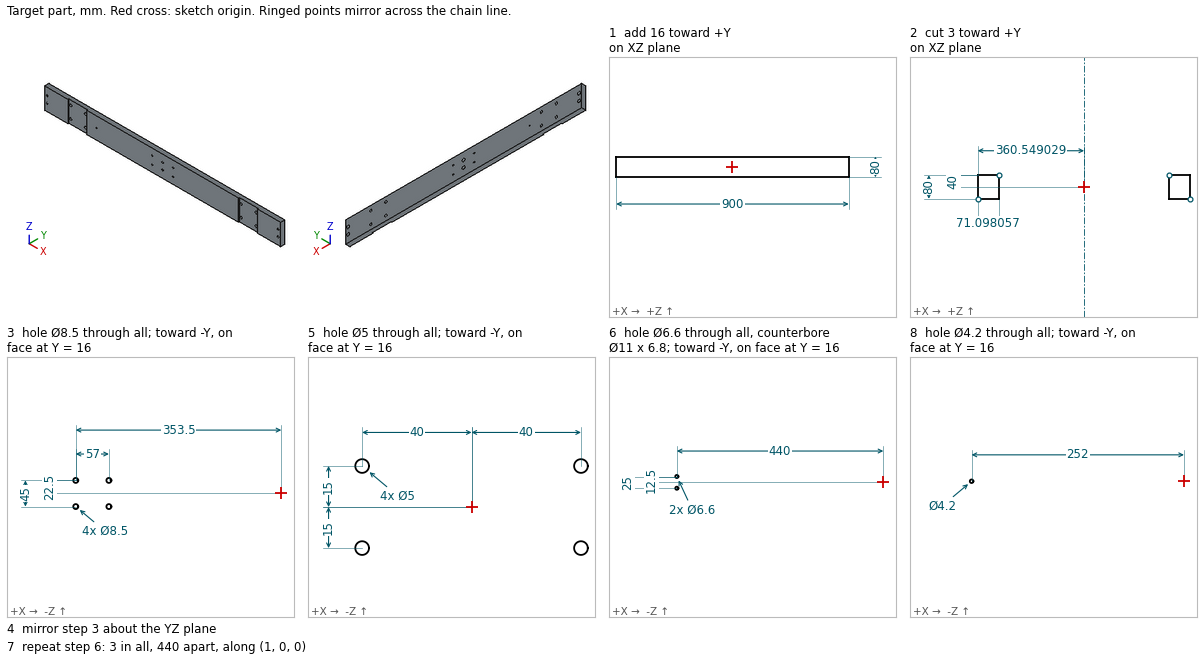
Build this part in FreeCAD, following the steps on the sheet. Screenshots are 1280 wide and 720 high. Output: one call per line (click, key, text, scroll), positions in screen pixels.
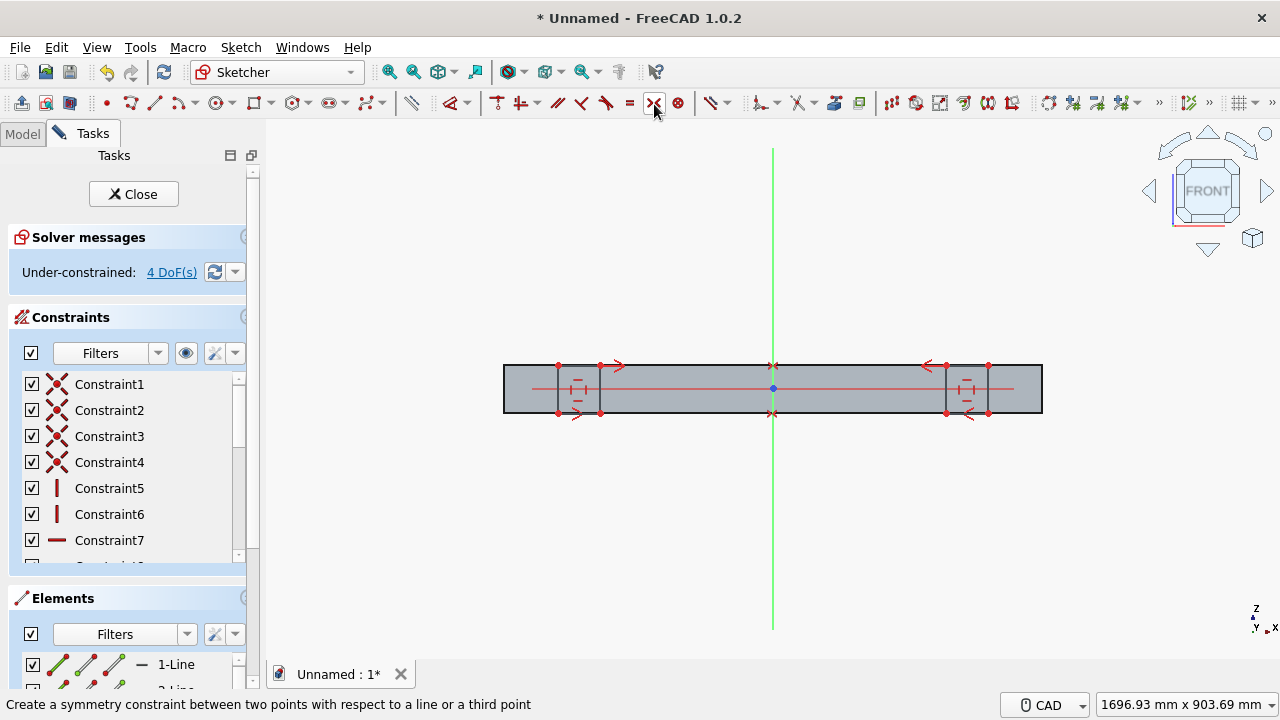
click(450, 104)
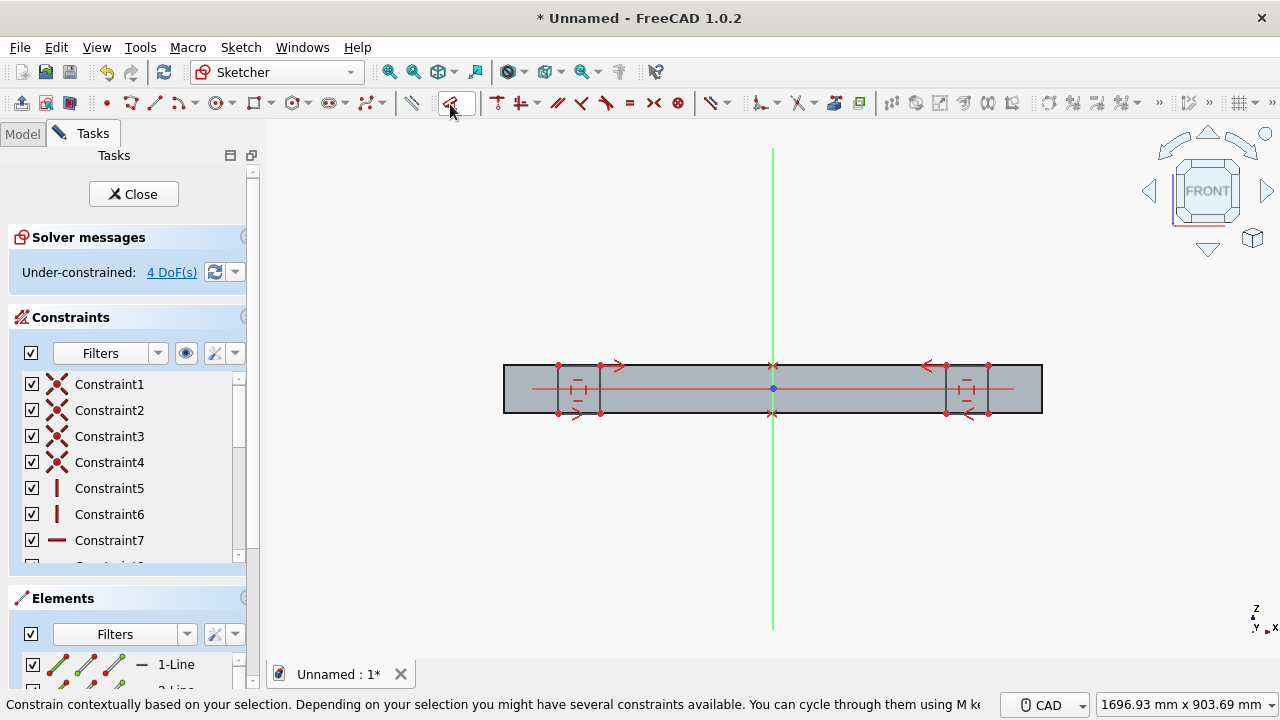
scroll(558, 400, up, 2)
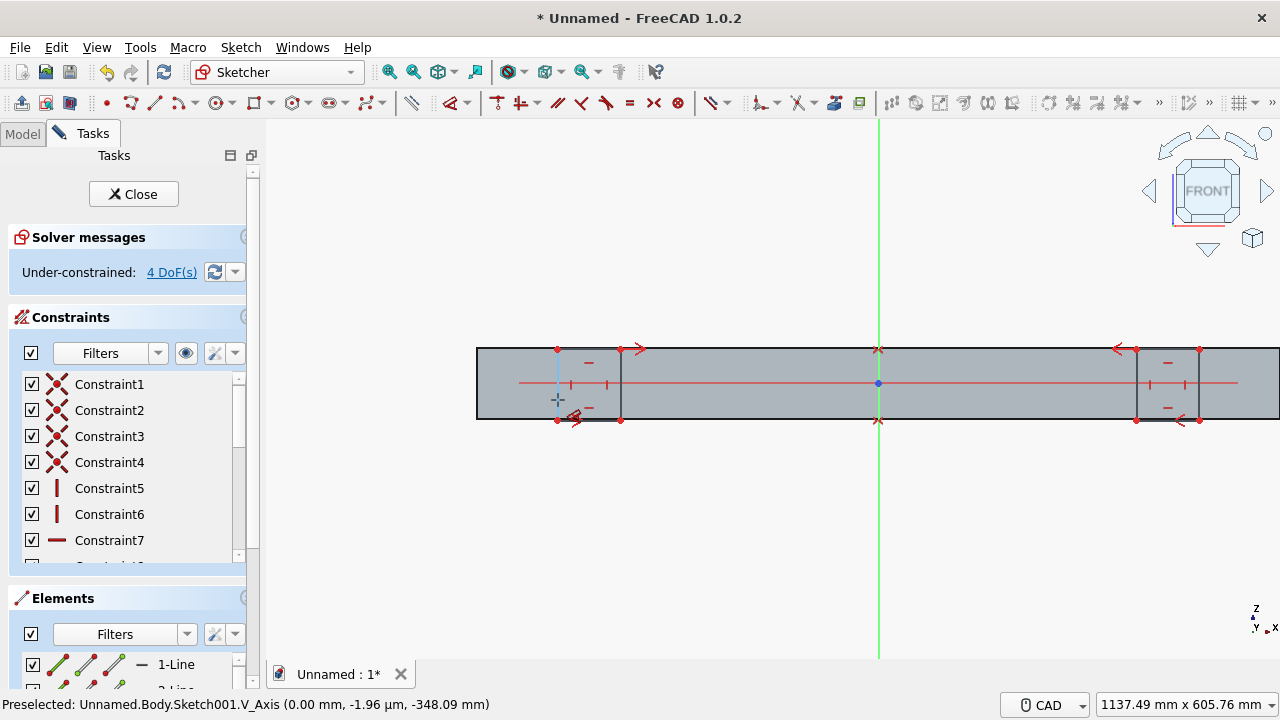
click(558, 399)
click(524, 368)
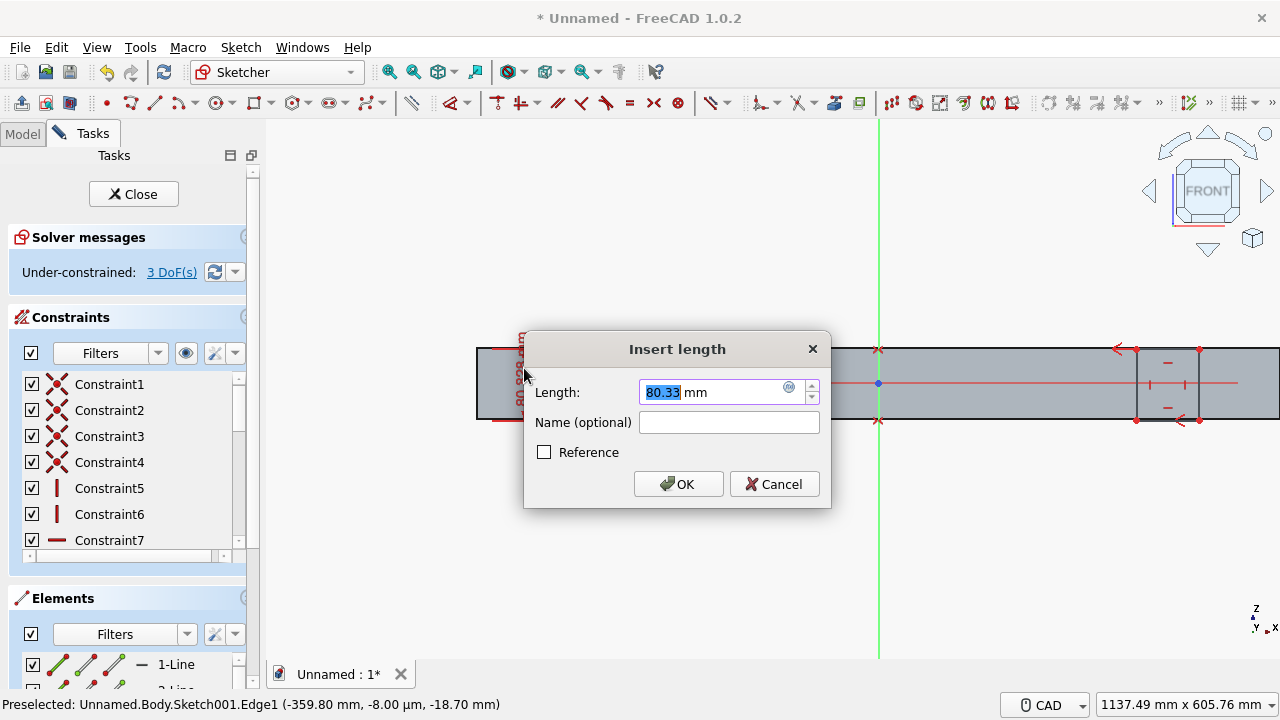
text(80)
key(Return)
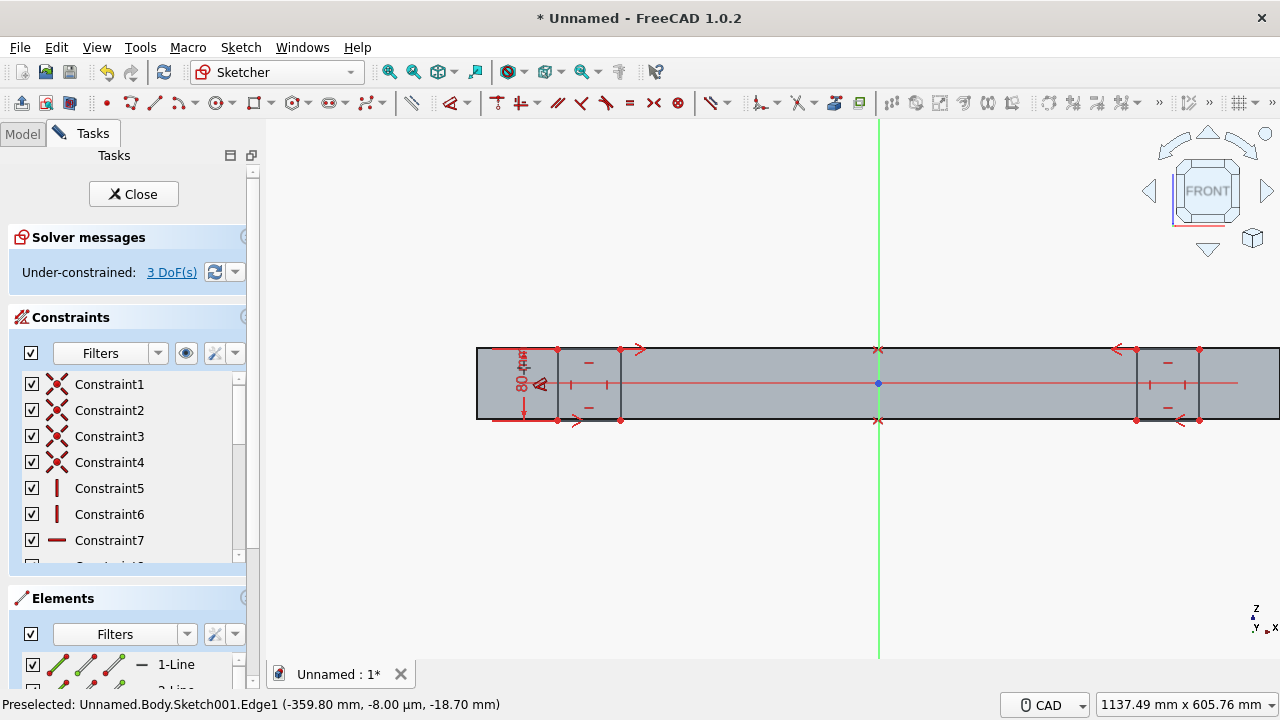
click(558, 349)
click(913, 366)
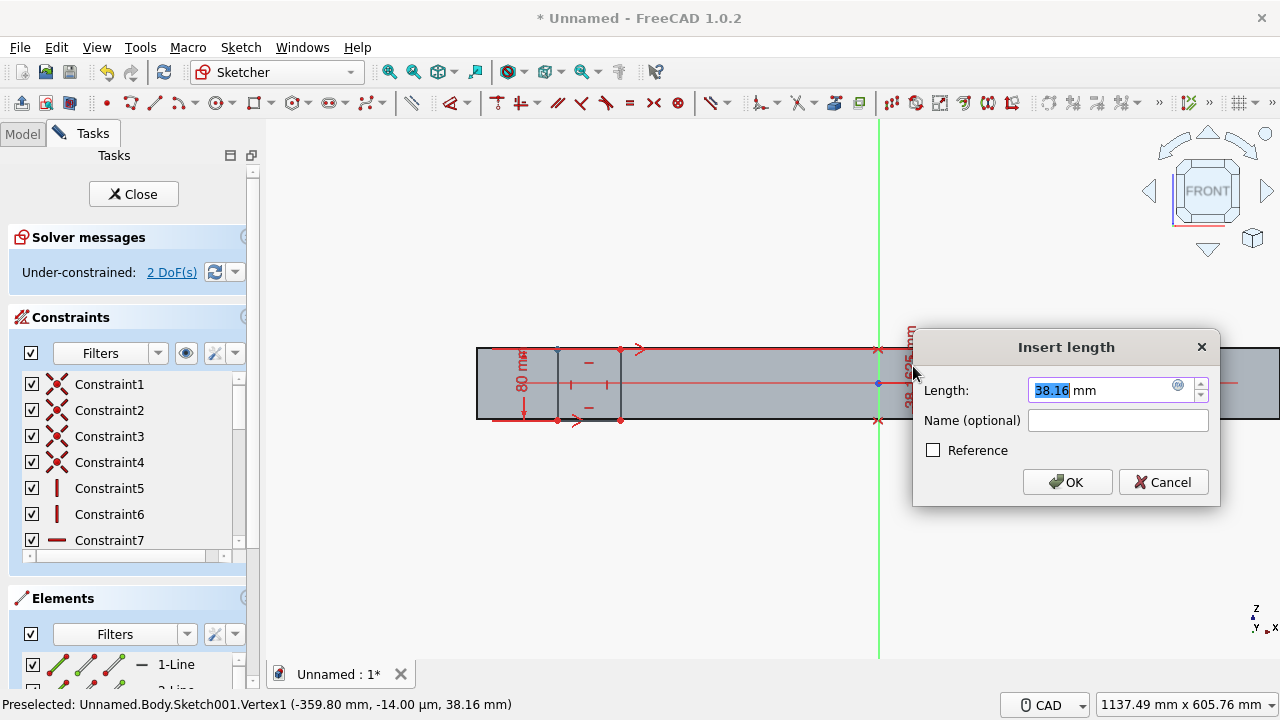
text(40)
key(Return)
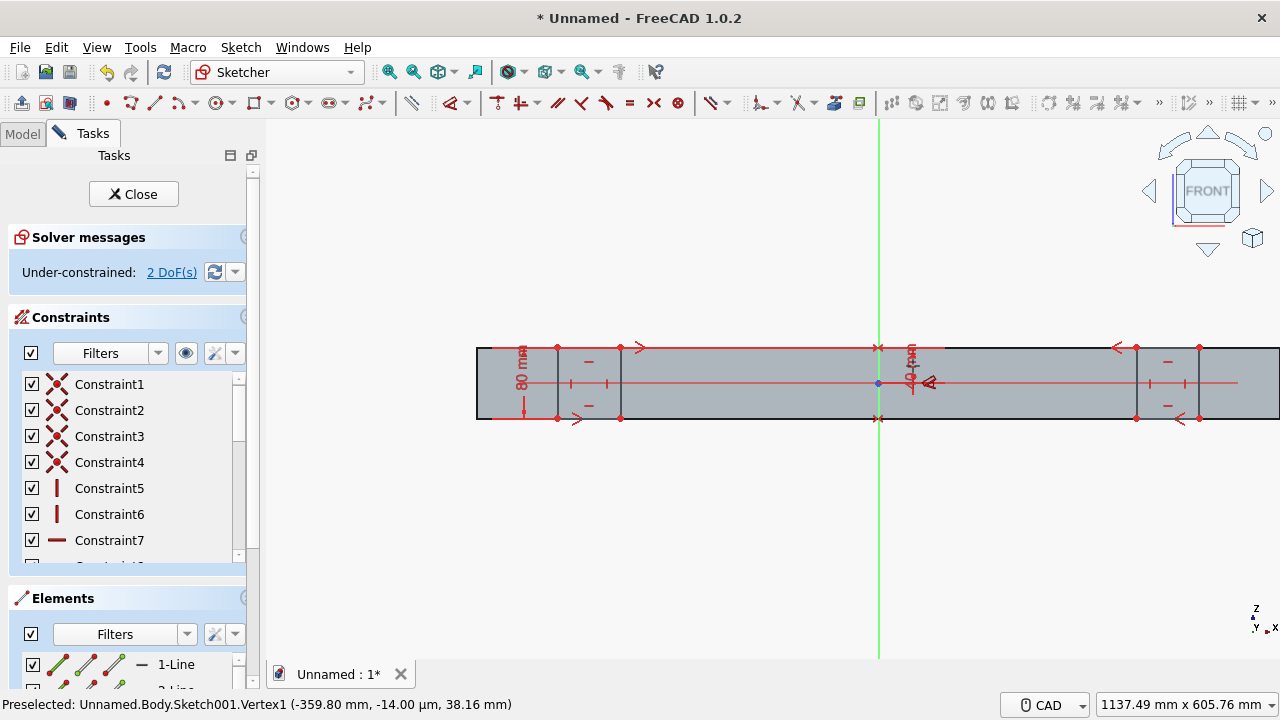
click(577, 419)
click(589, 453)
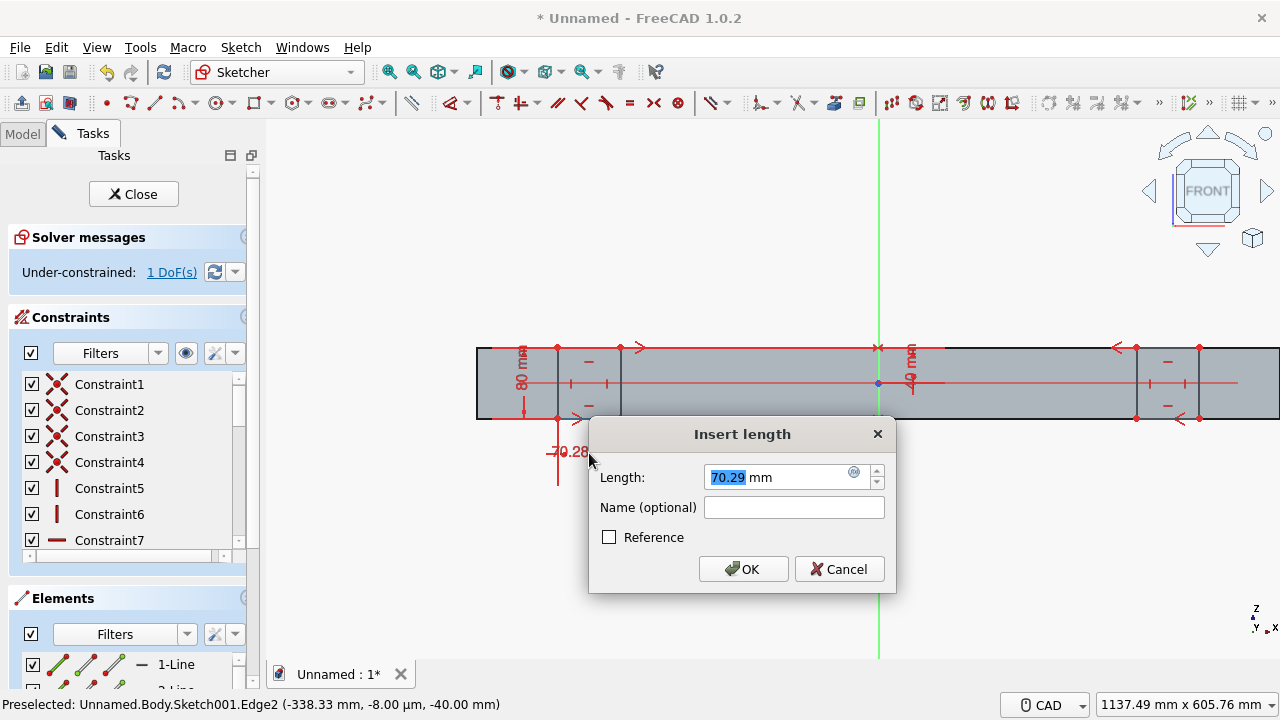
text(71.098057)
key(Return)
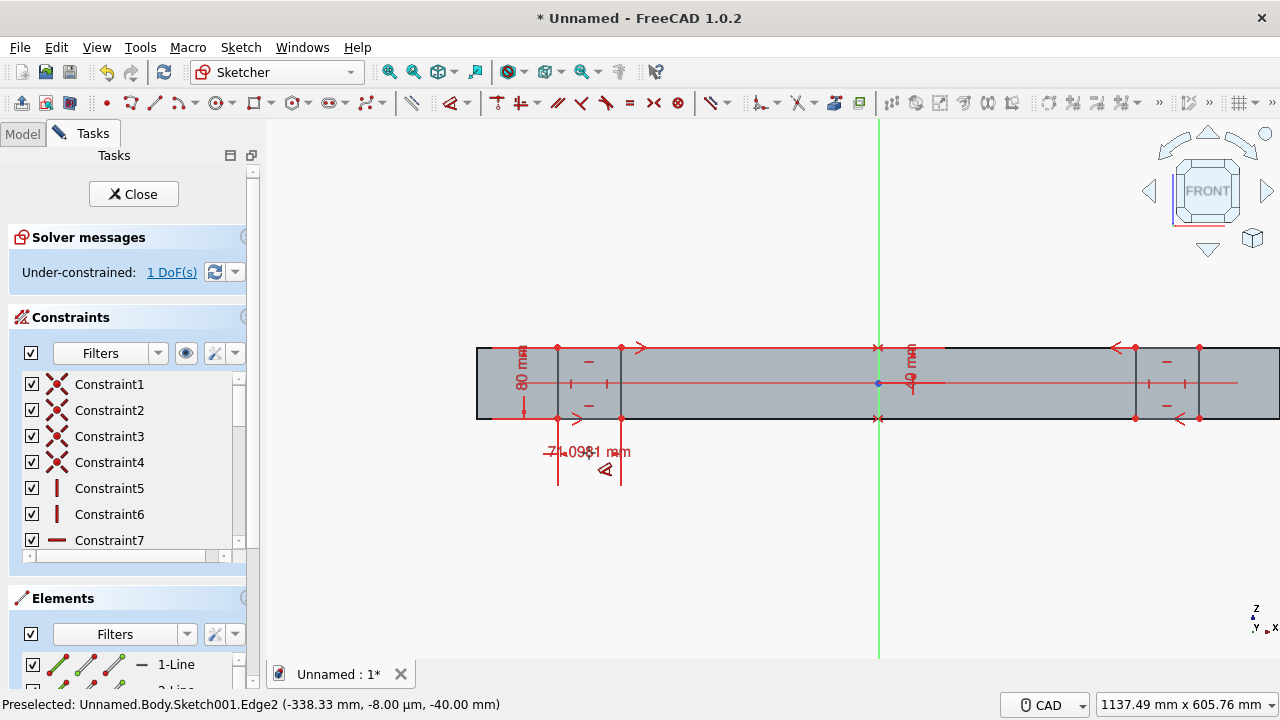
click(558, 348)
click(718, 314)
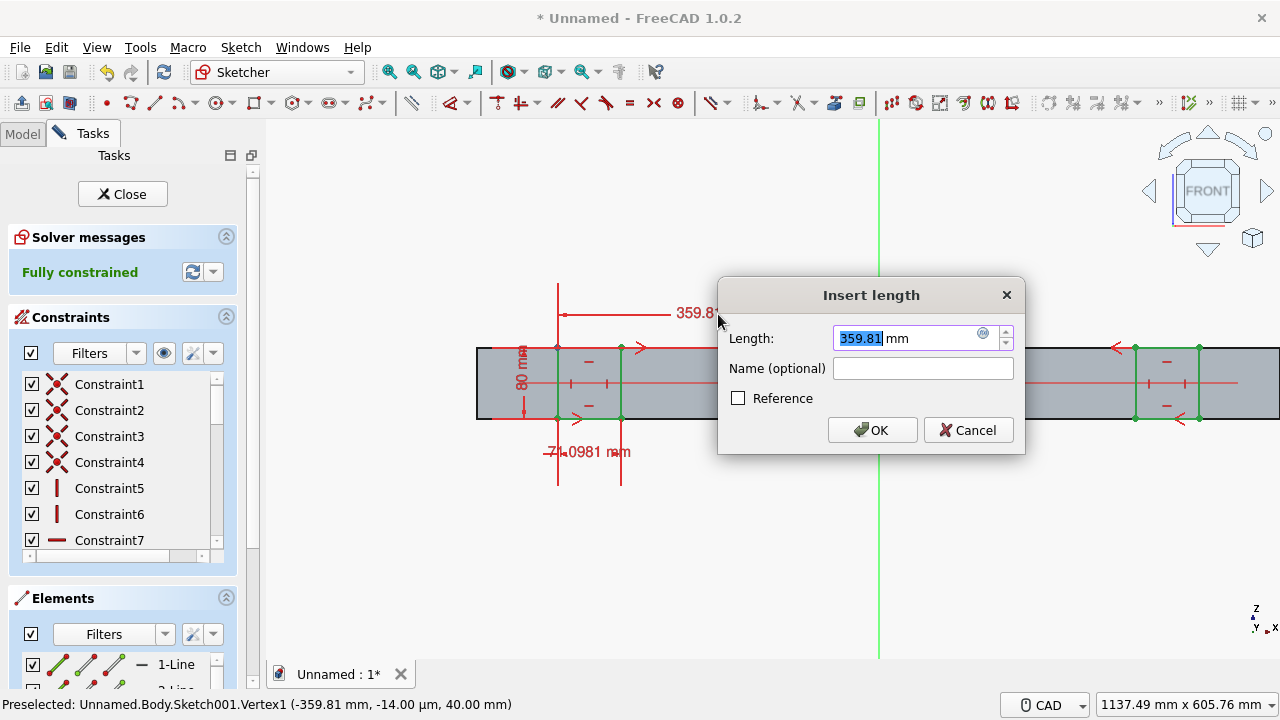
text(360.549029)
key(Return)
key(Escape)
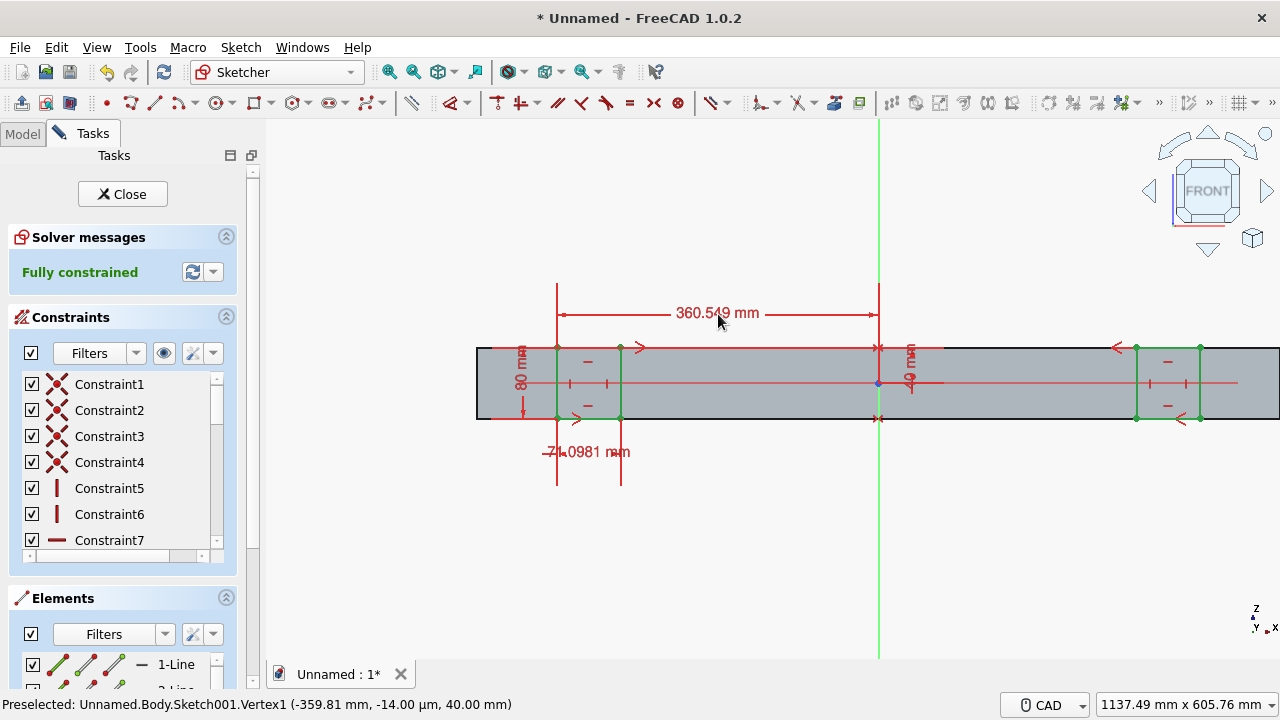
click(123, 194)